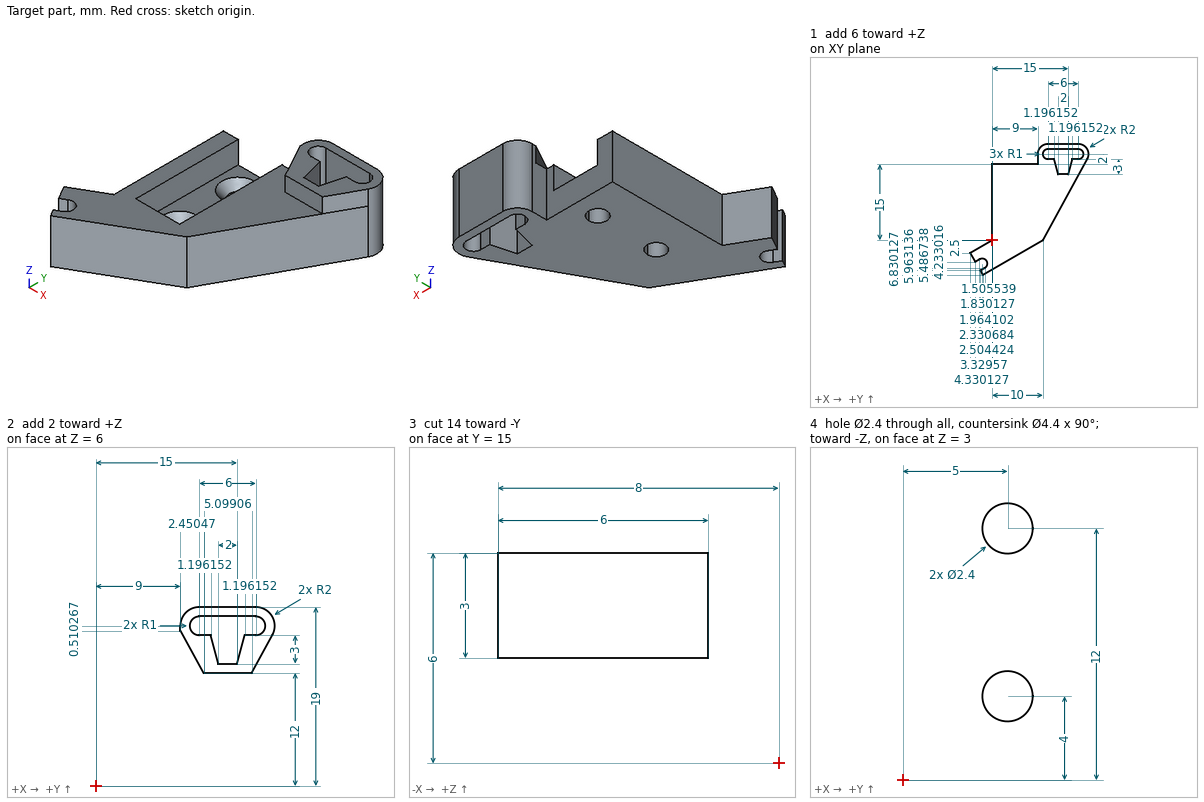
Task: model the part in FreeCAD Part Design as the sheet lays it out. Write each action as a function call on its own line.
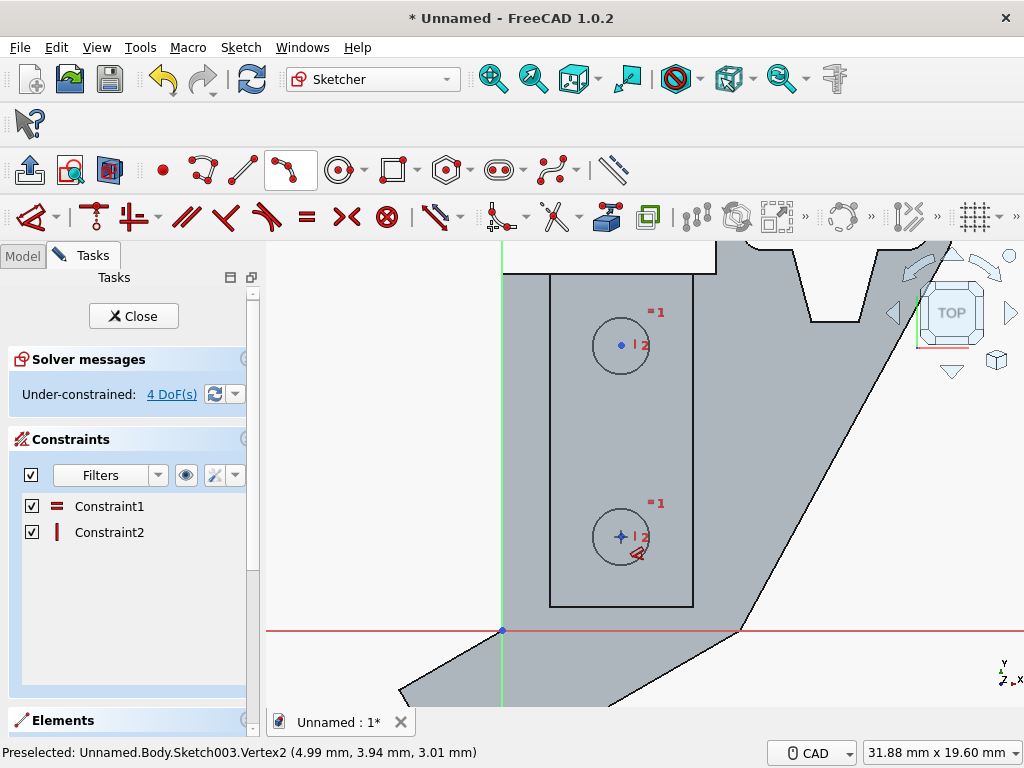
click(641, 326)
click(664, 303)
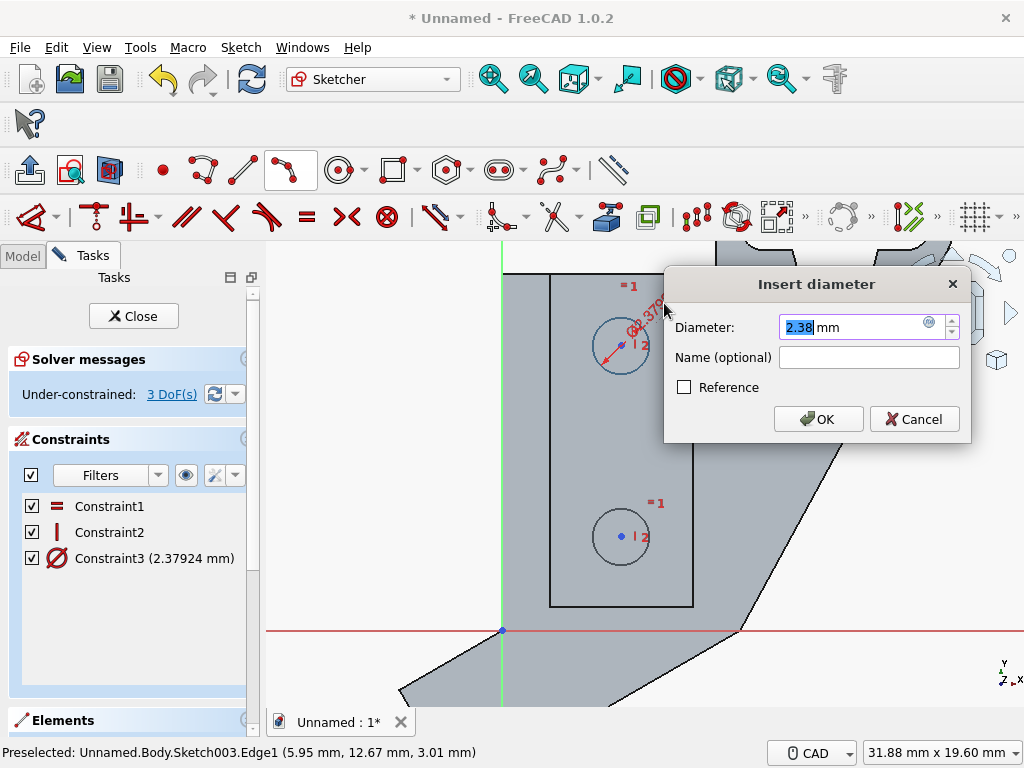
text(2.4)
key(Return)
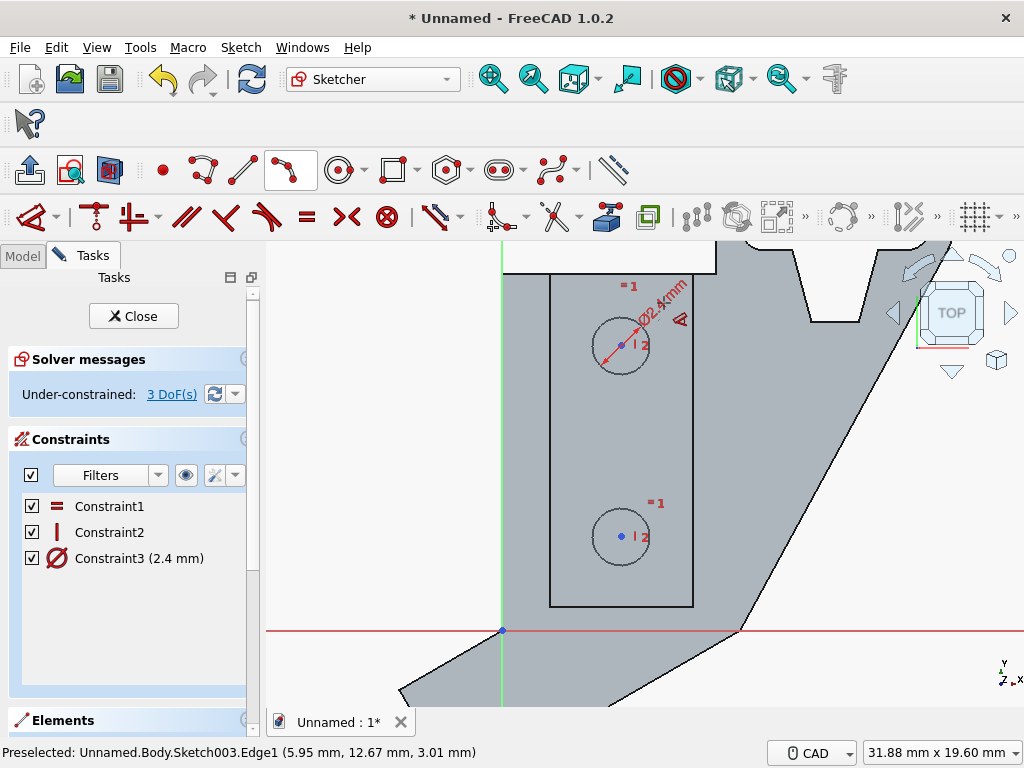
click(621, 346)
click(562, 665)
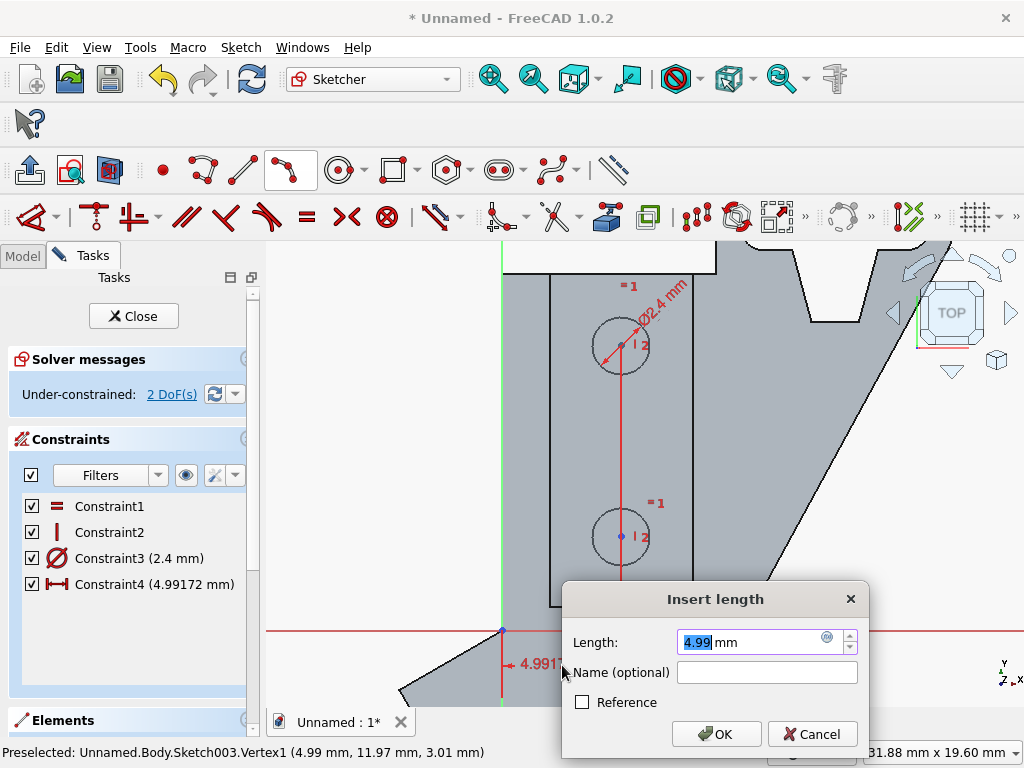
text(5)
key(Return)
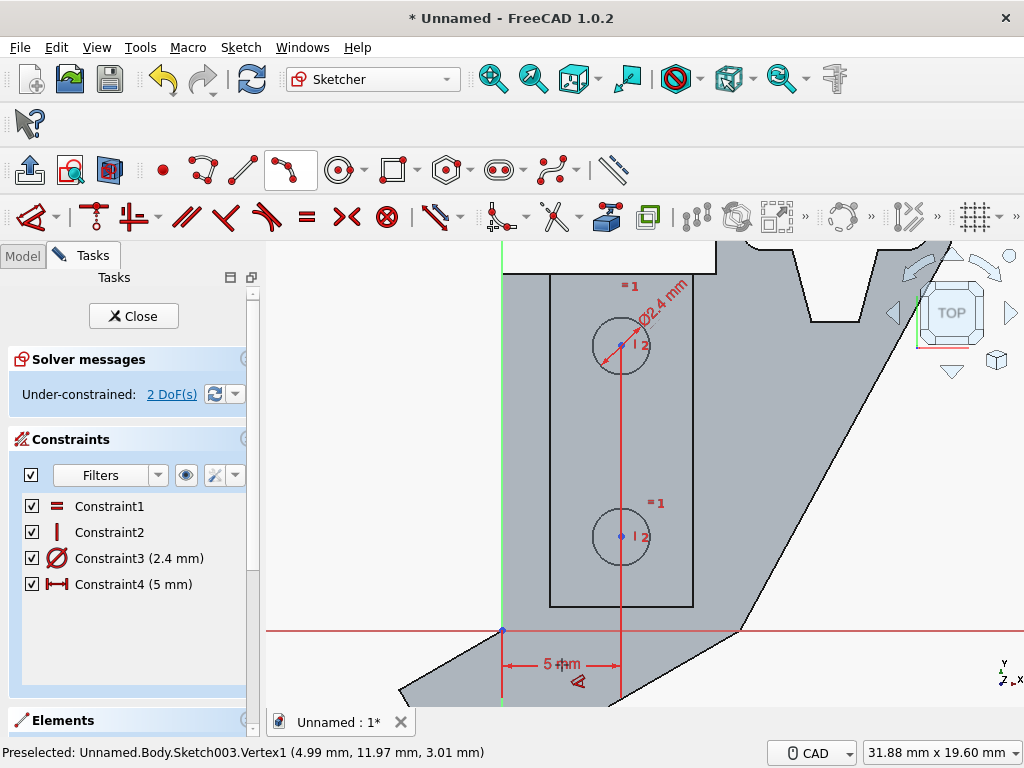
click(621, 537)
click(468, 584)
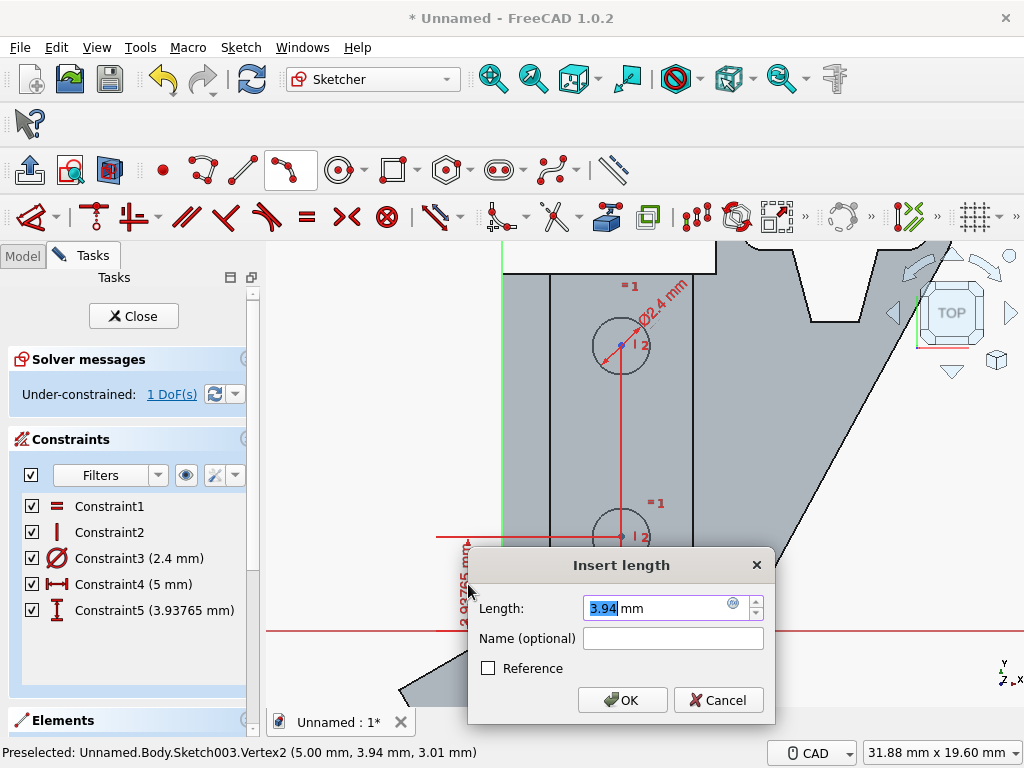
text(4)
key(Return)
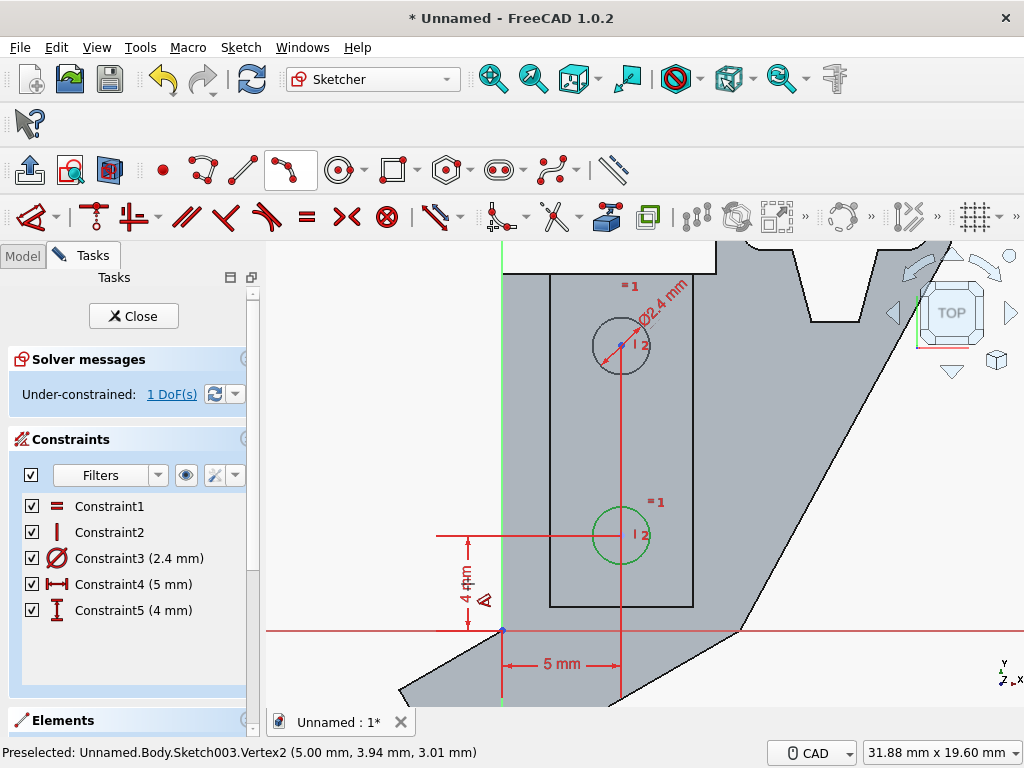
click(621, 346)
click(468, 488)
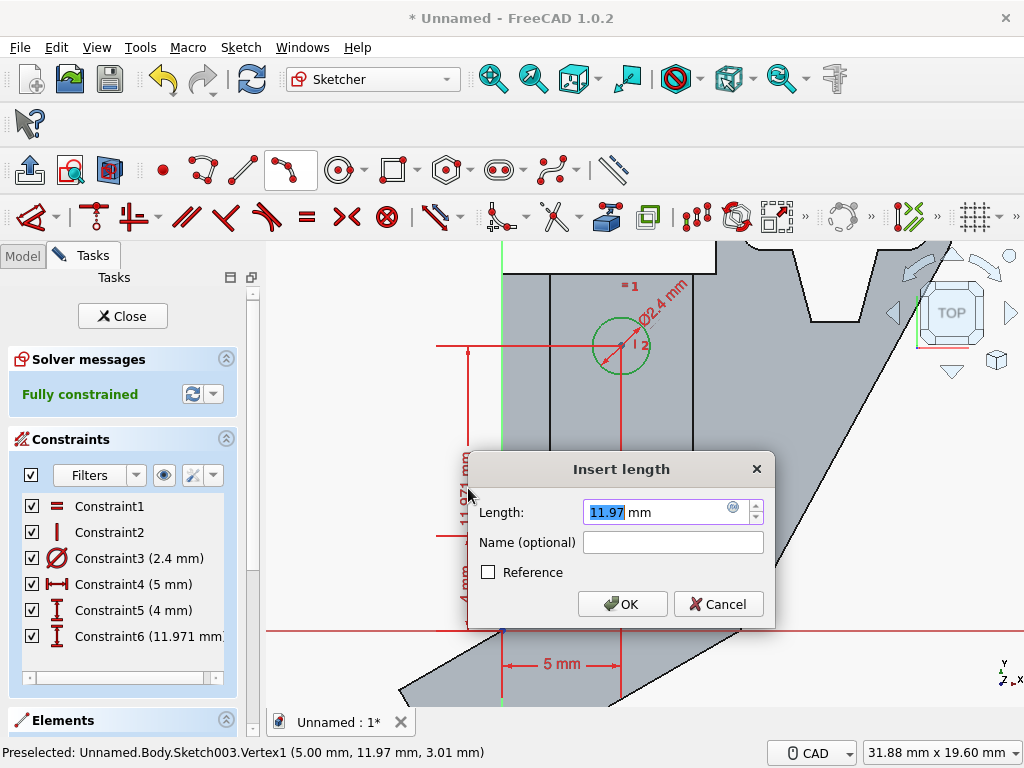
text(12)
key(Return)
key(Escape)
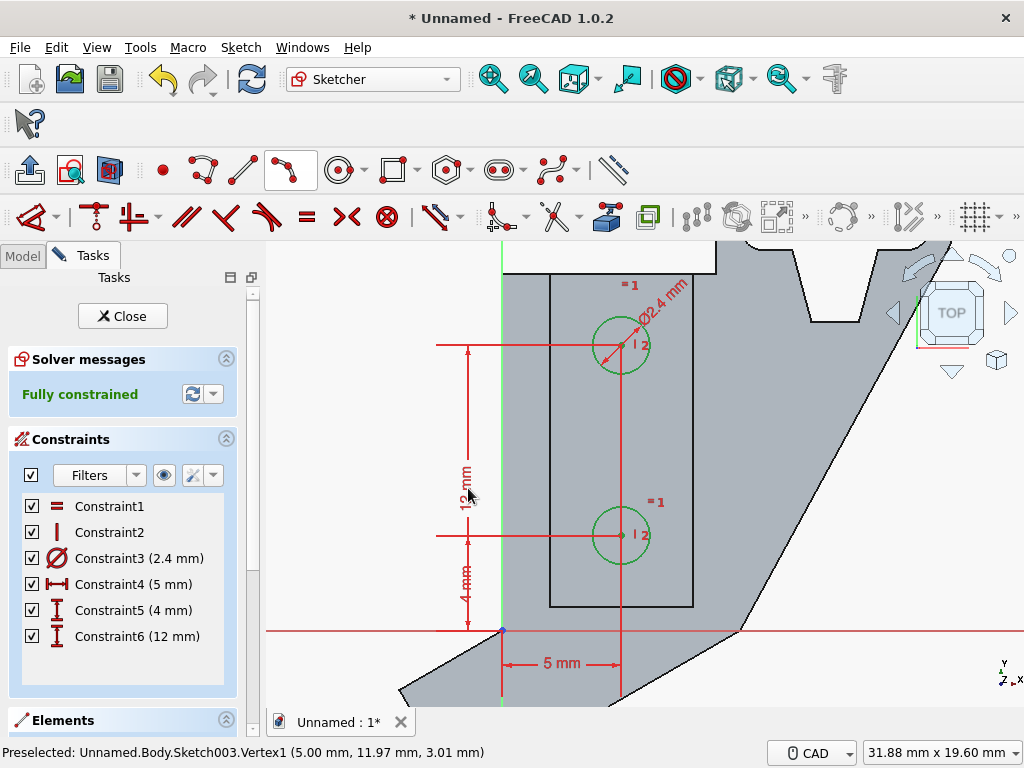
click(123, 316)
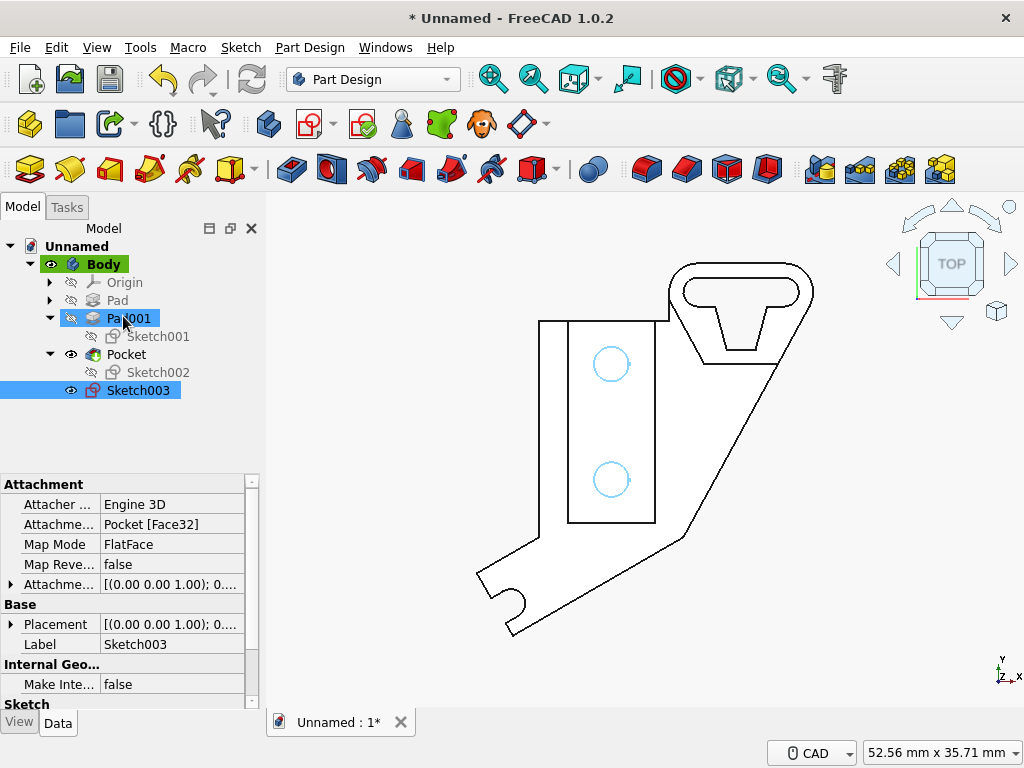
click(332, 170)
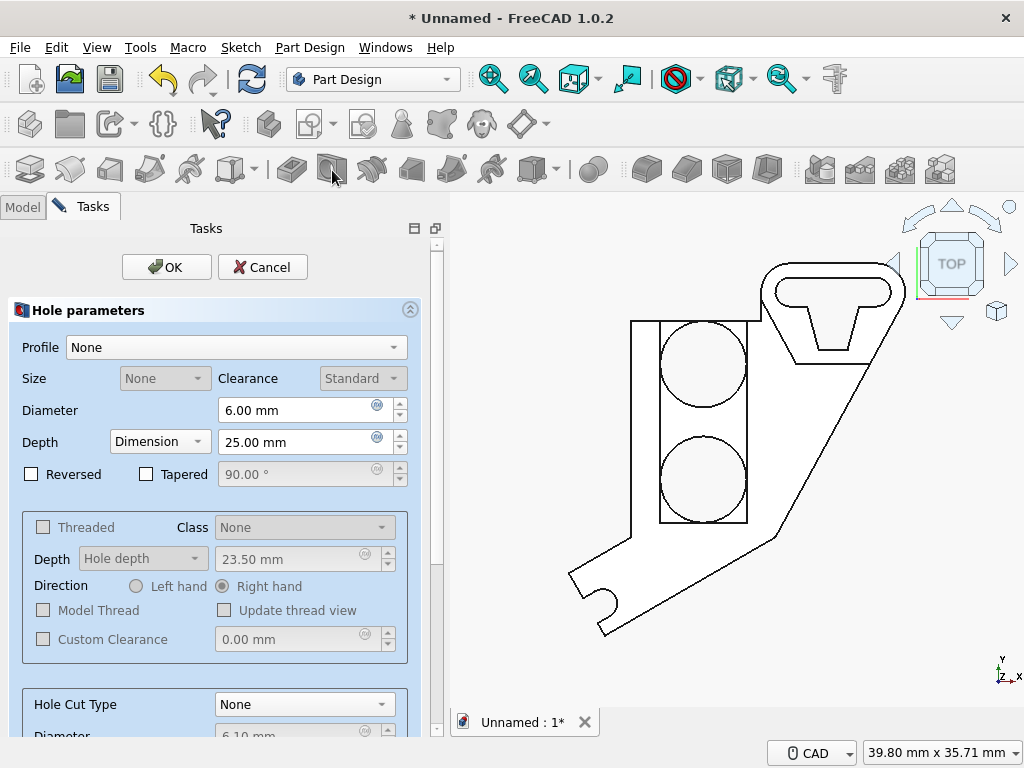
triple_click(305, 410)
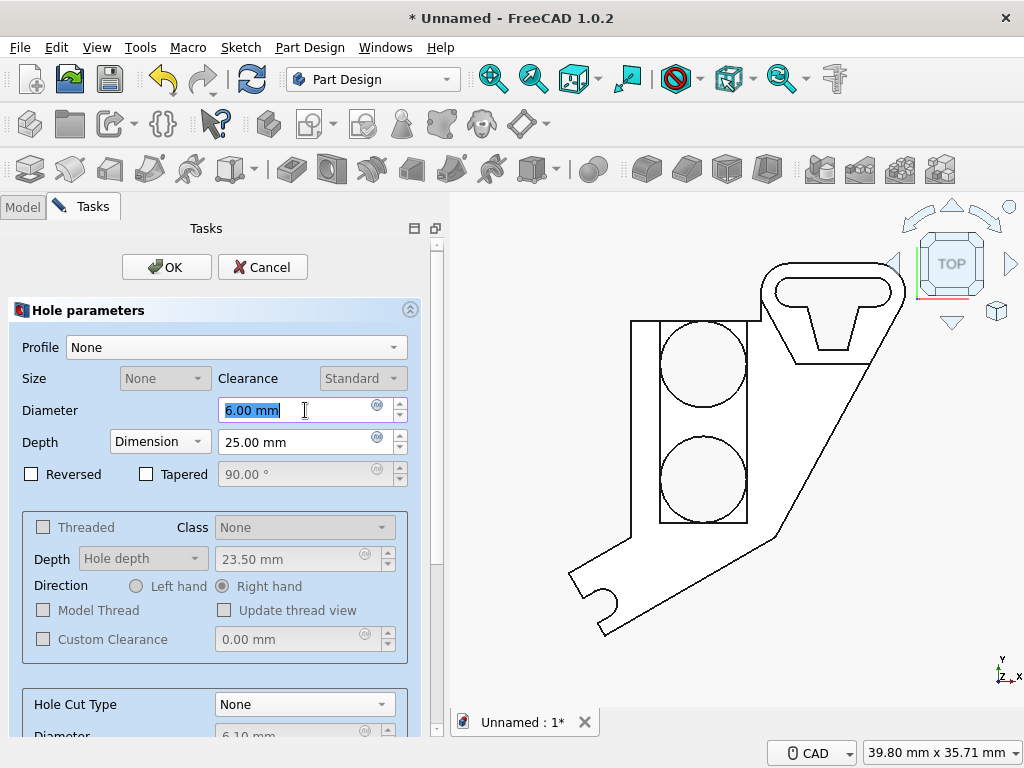
text(2.4)
key(Tab)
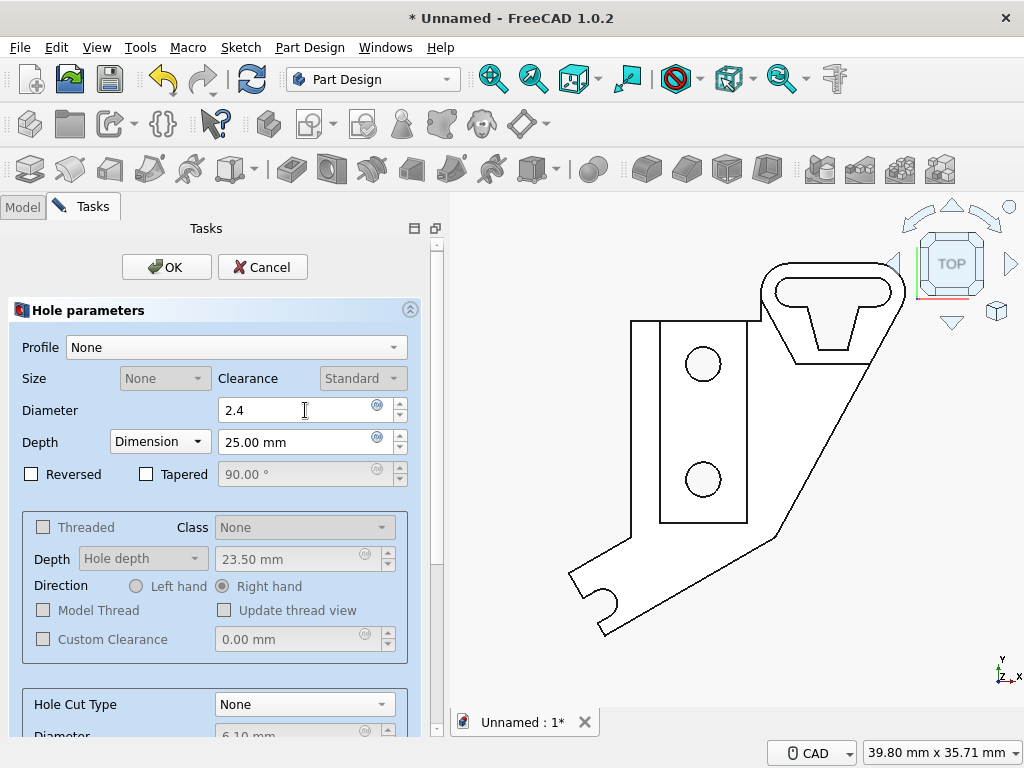
click(161, 442)